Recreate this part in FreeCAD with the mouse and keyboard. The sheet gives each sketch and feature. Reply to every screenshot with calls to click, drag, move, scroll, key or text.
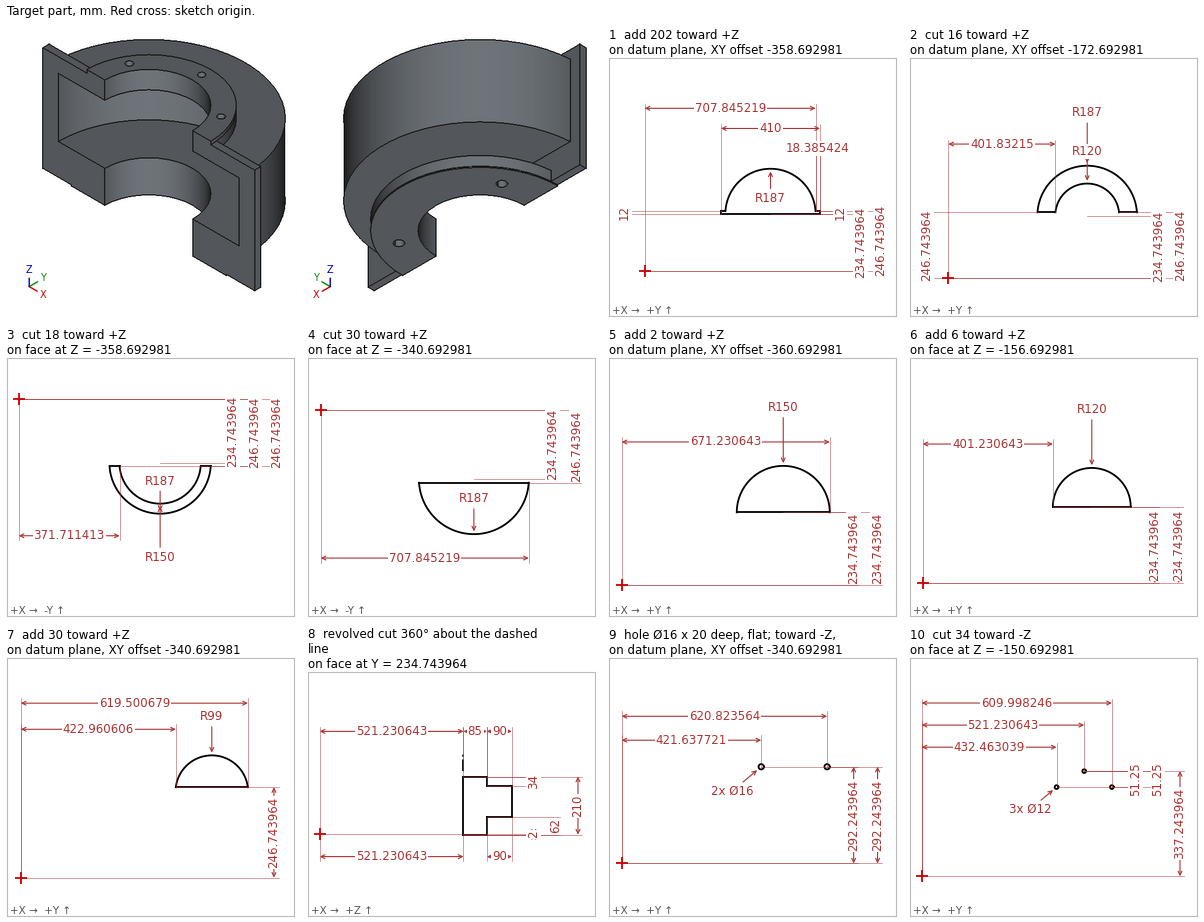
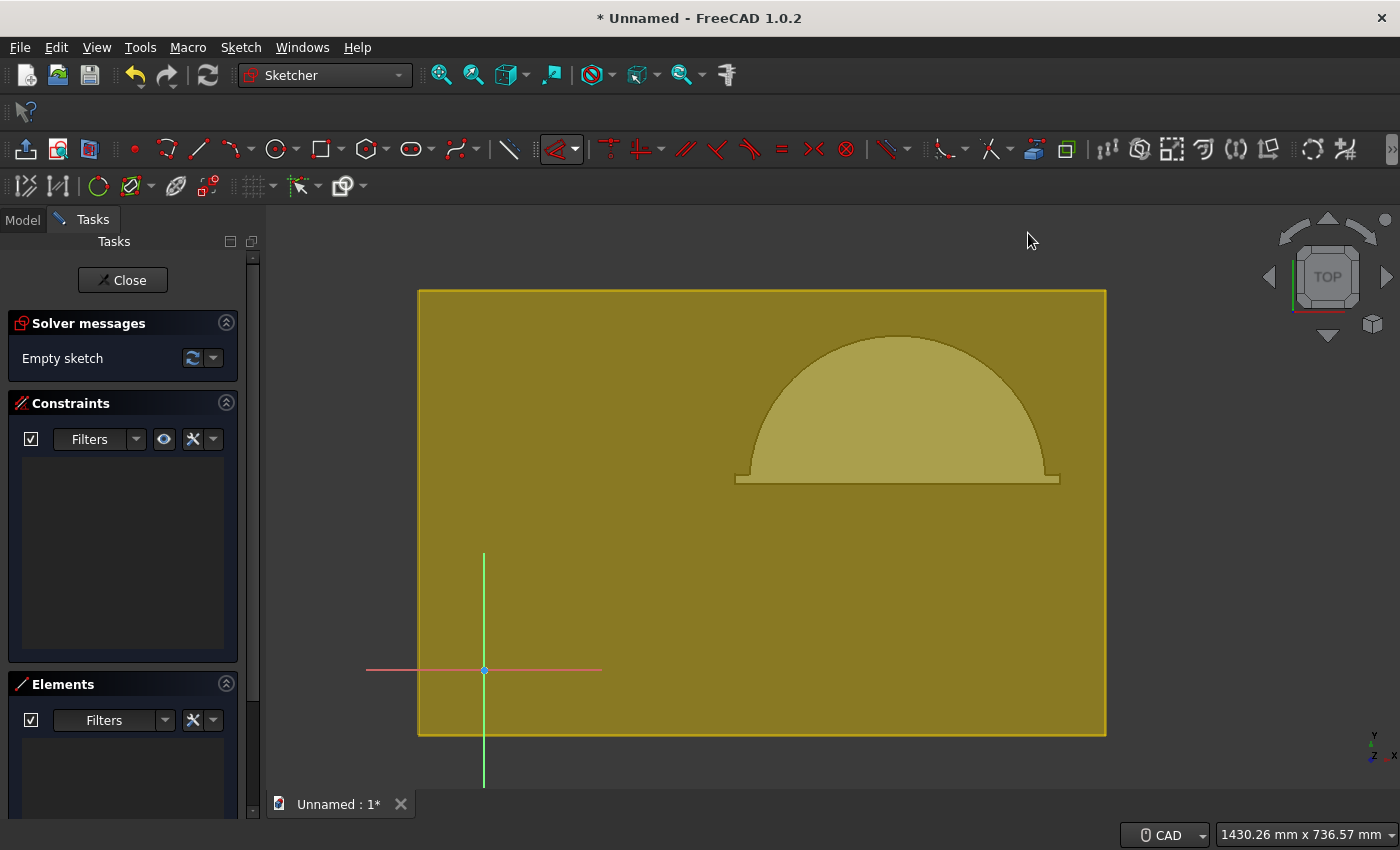
click(200, 150)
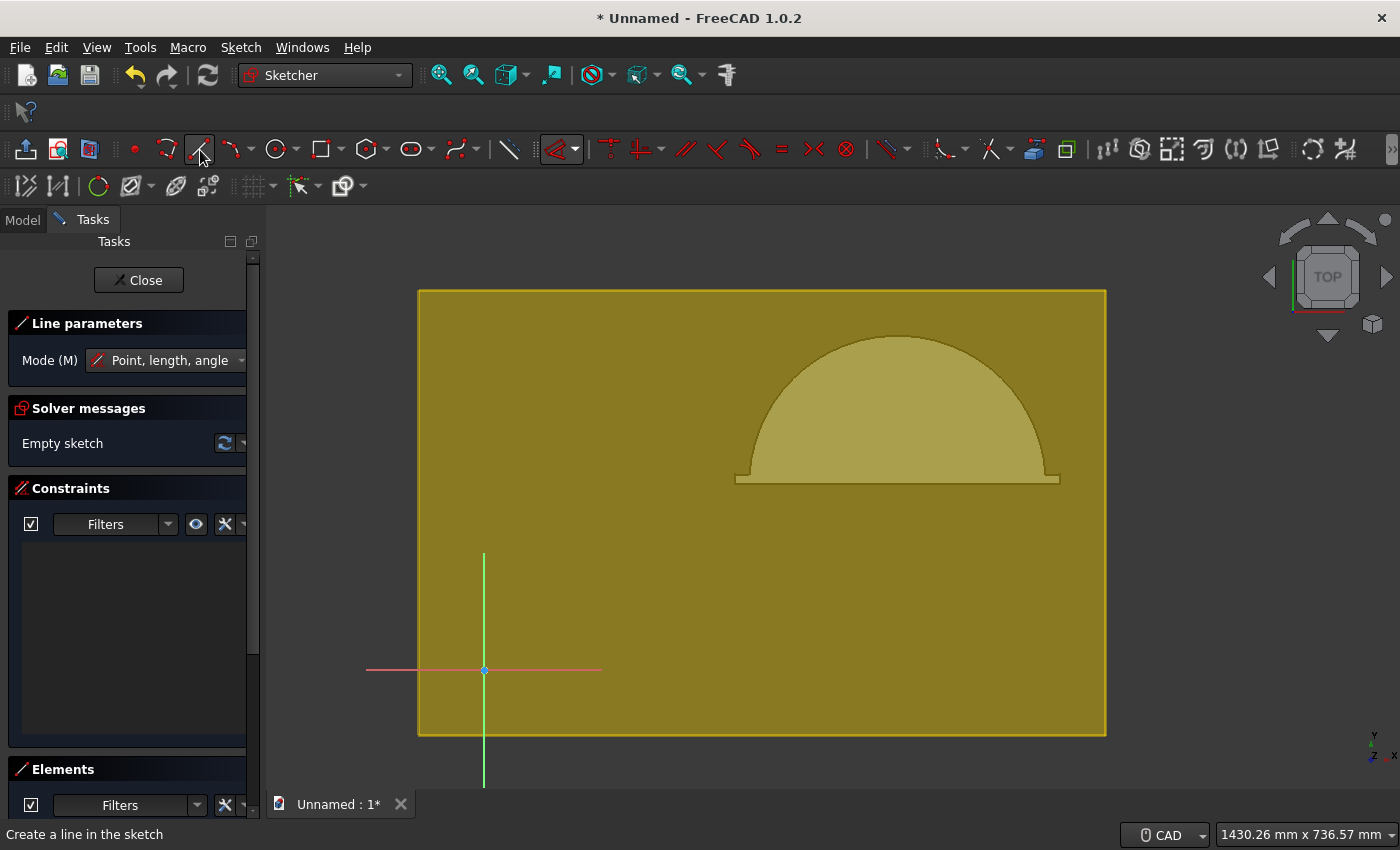
click(992, 474)
click(1045, 474)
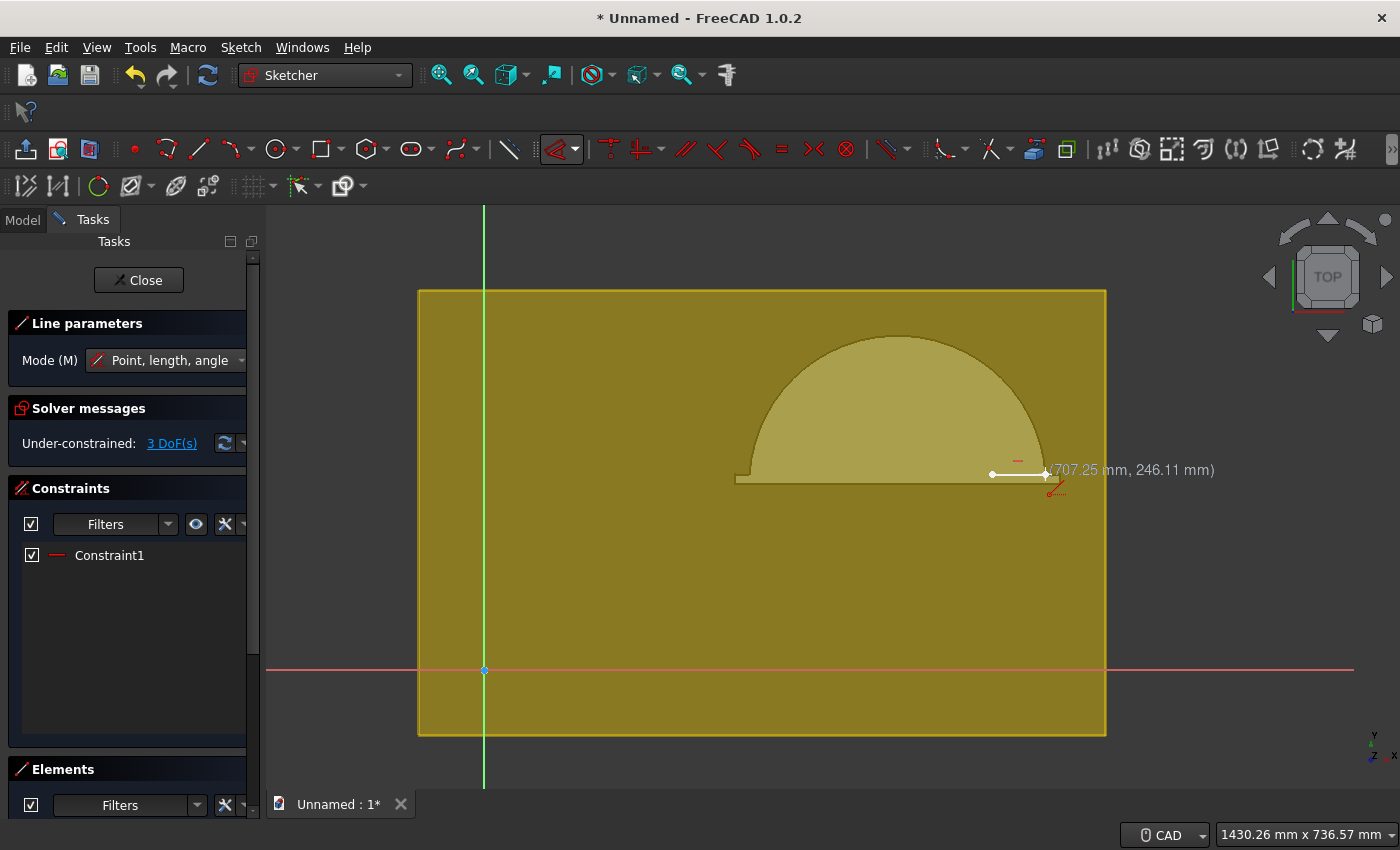
click(750, 474)
click(803, 474)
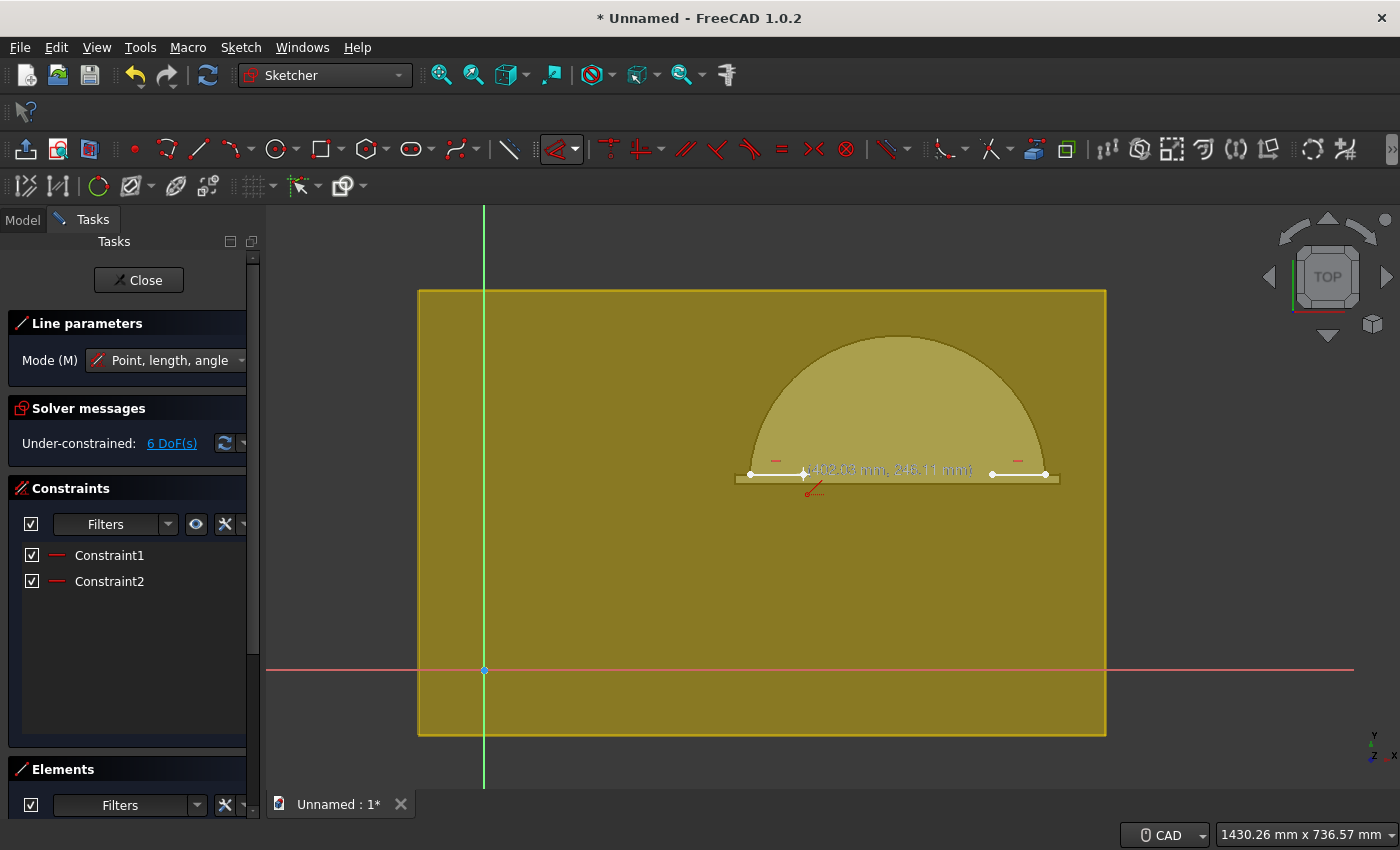
key(g)
key(3)
key(a)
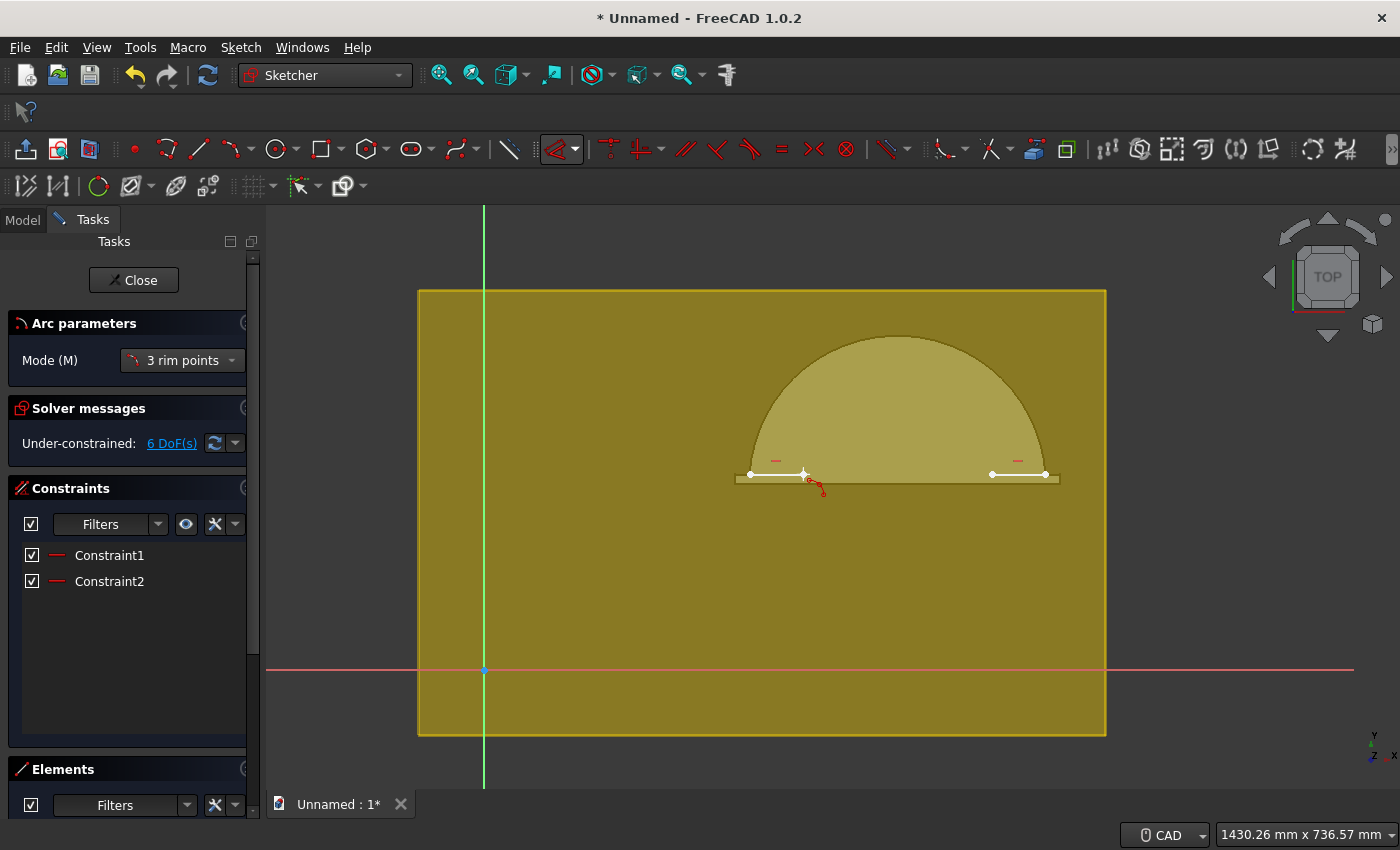
click(1045, 475)
click(750, 475)
click(898, 336)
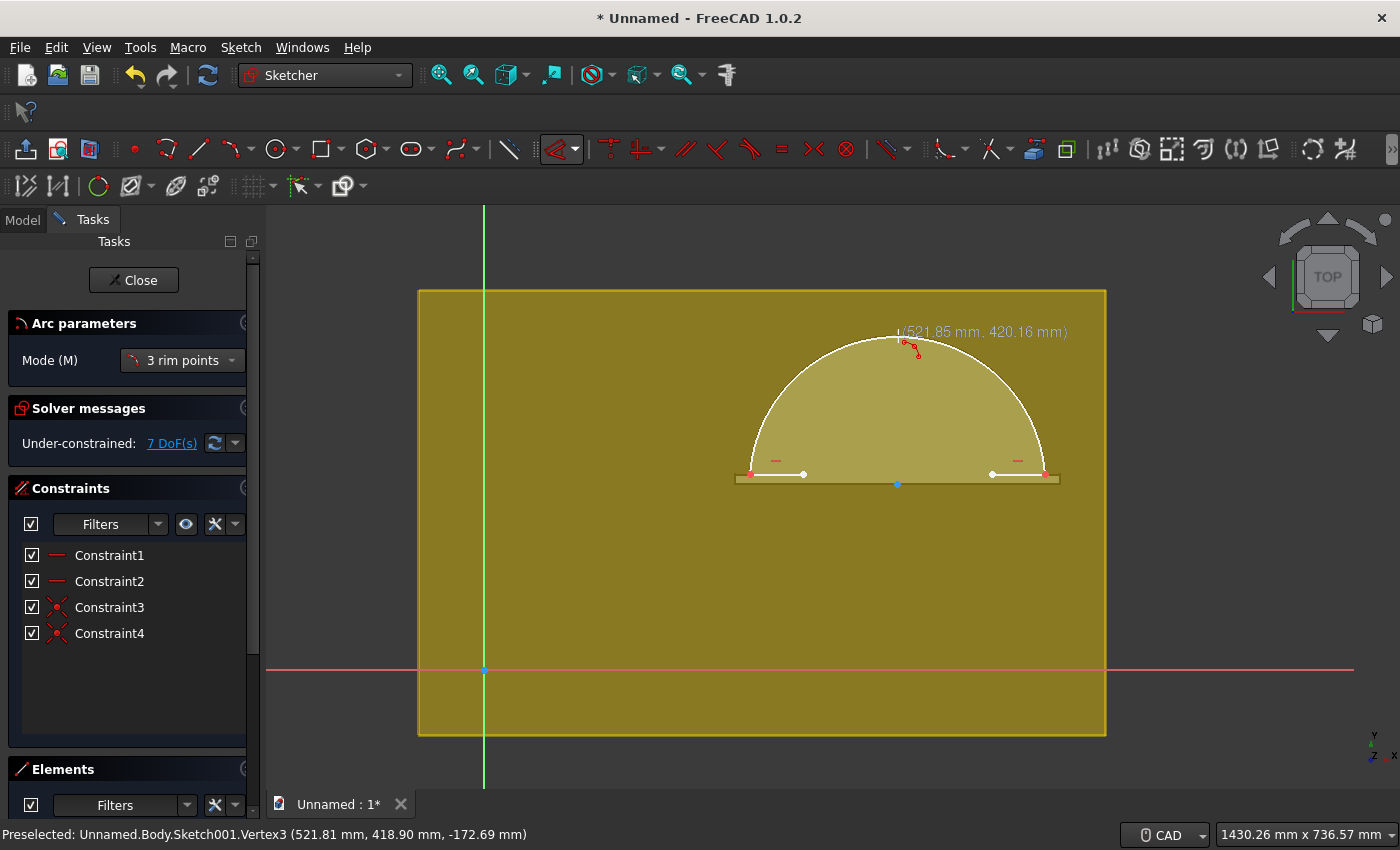
click(803, 475)
click(992, 475)
click(898, 389)
key(Escape)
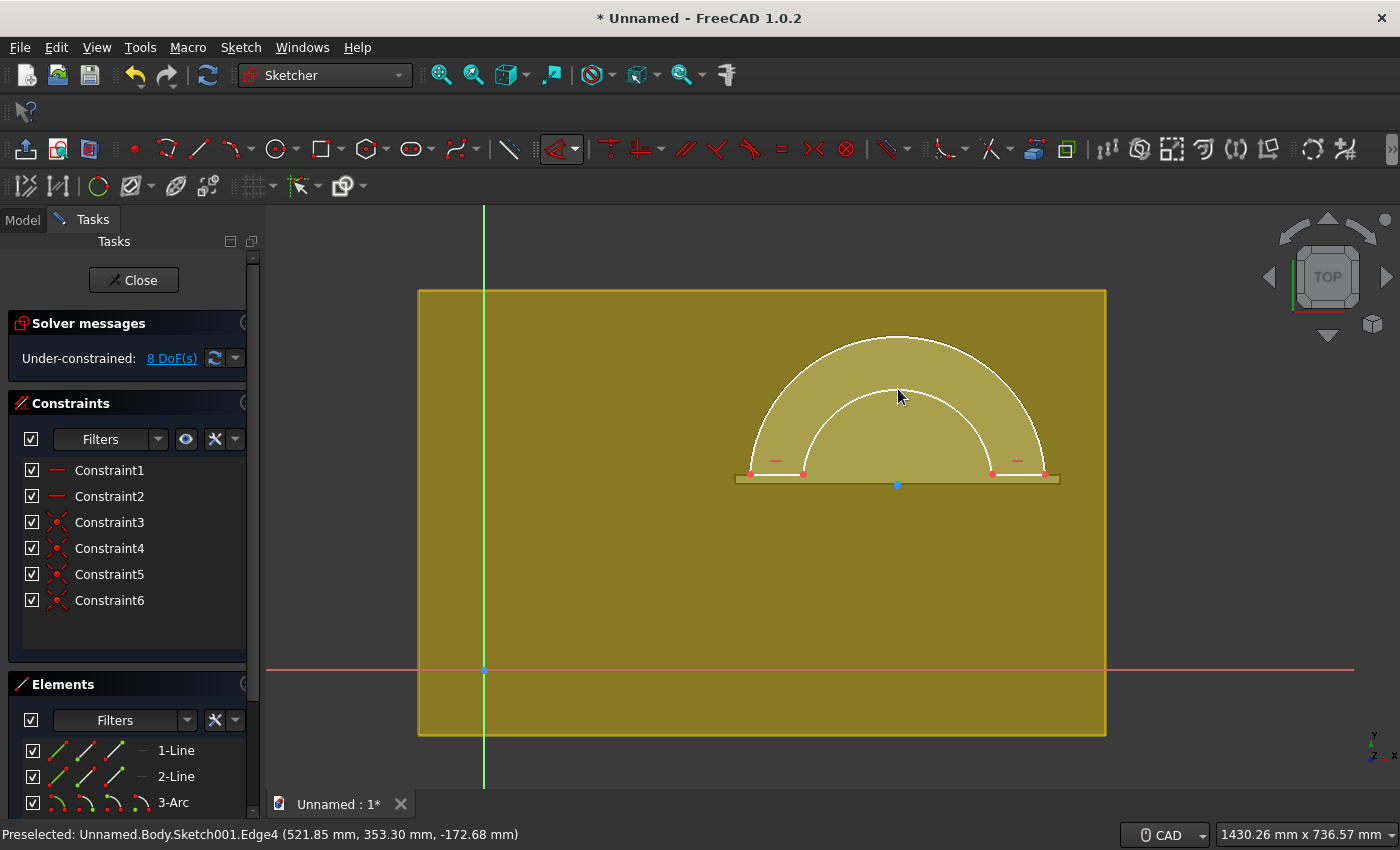
click(981, 363)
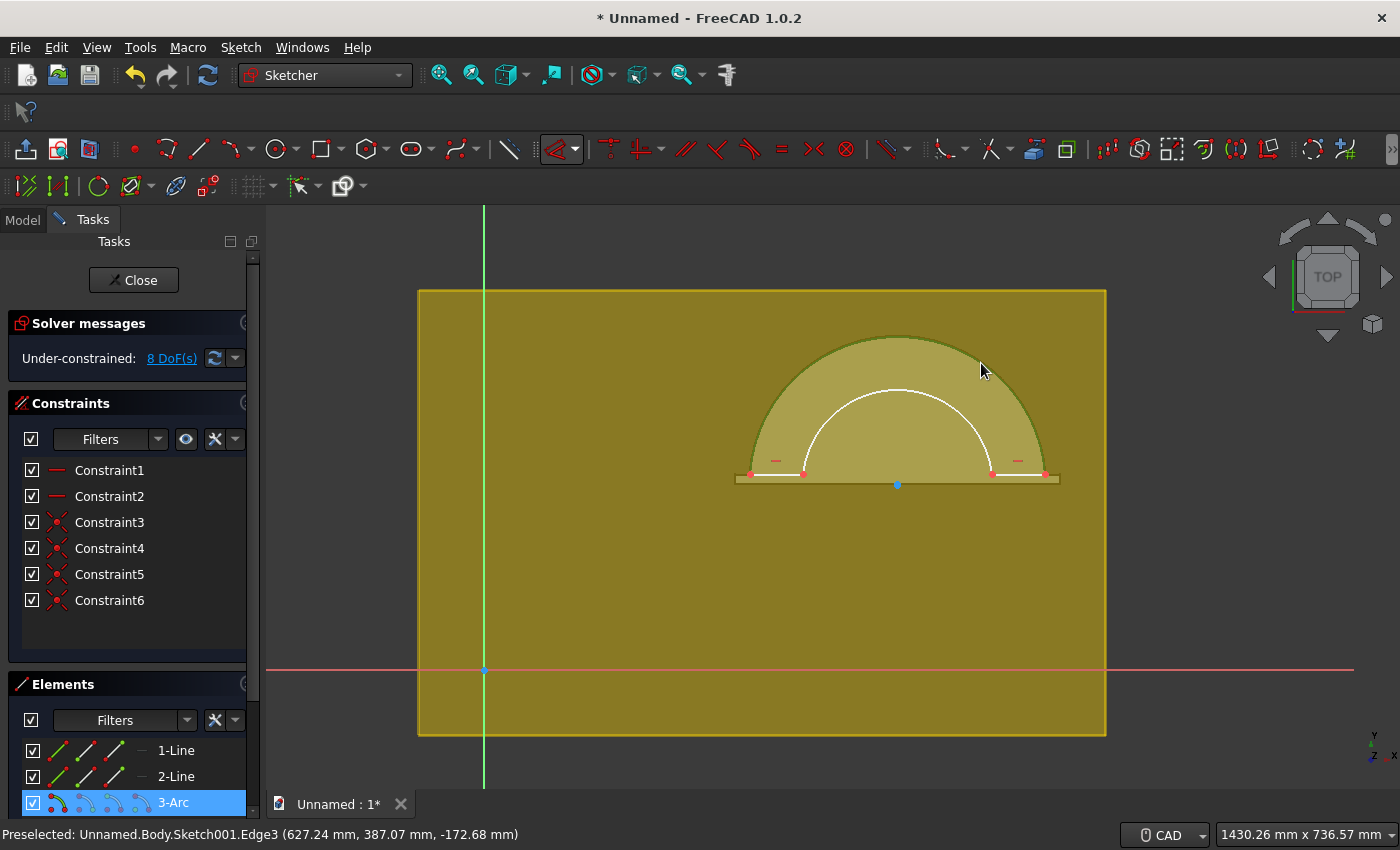
click(950, 406)